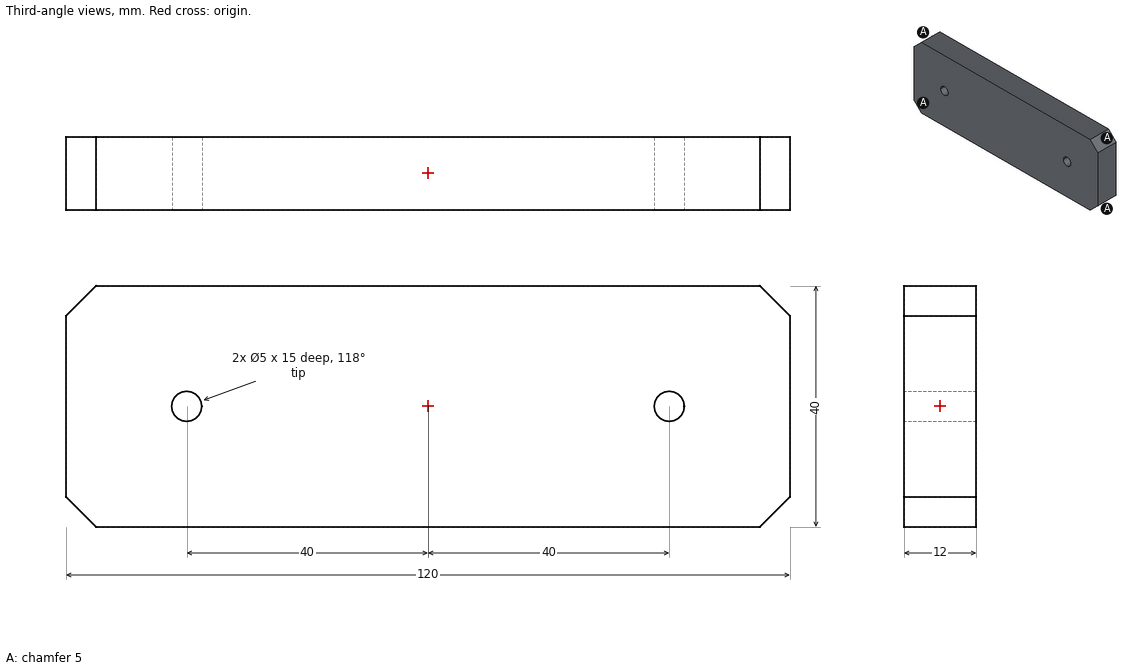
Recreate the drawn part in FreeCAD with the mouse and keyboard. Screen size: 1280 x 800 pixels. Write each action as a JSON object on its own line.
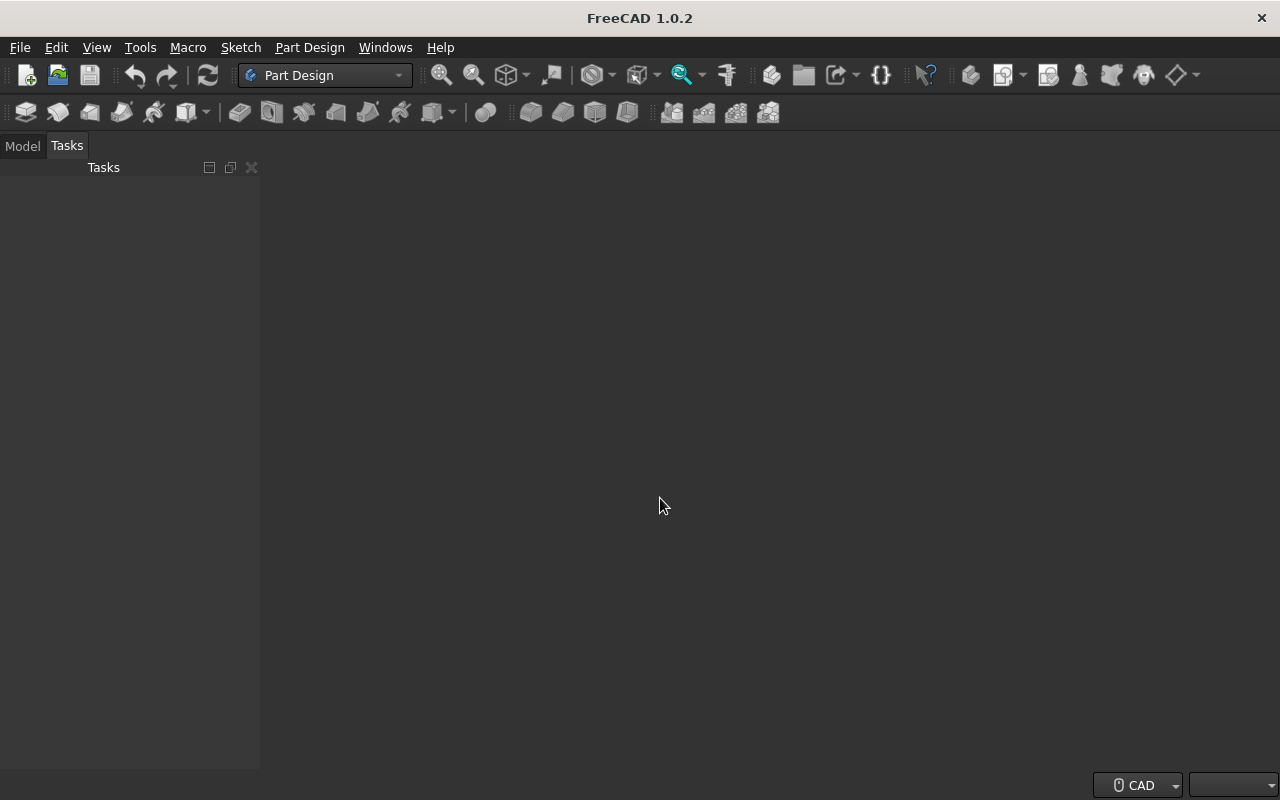
{"action": "left_click", "coordinate": [26, 76]}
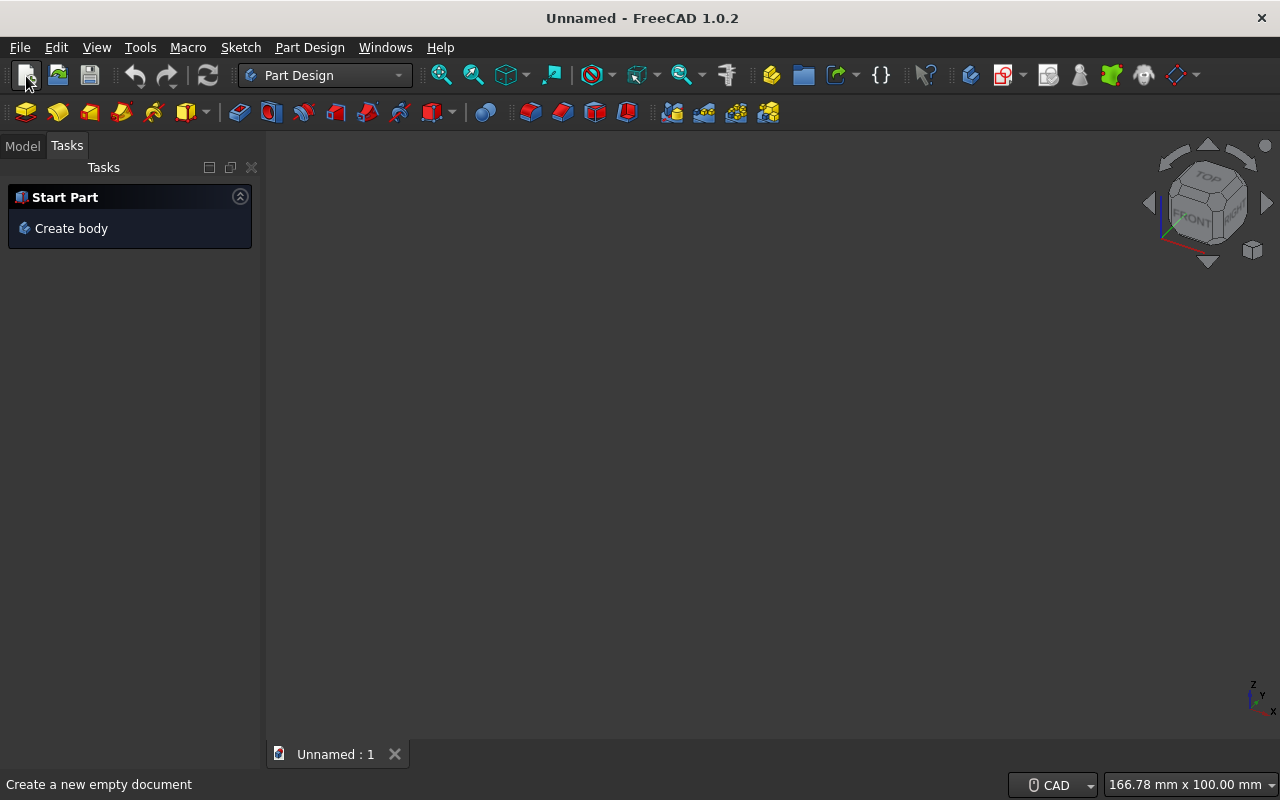
{"action": "left_click", "coordinate": [1004, 76]}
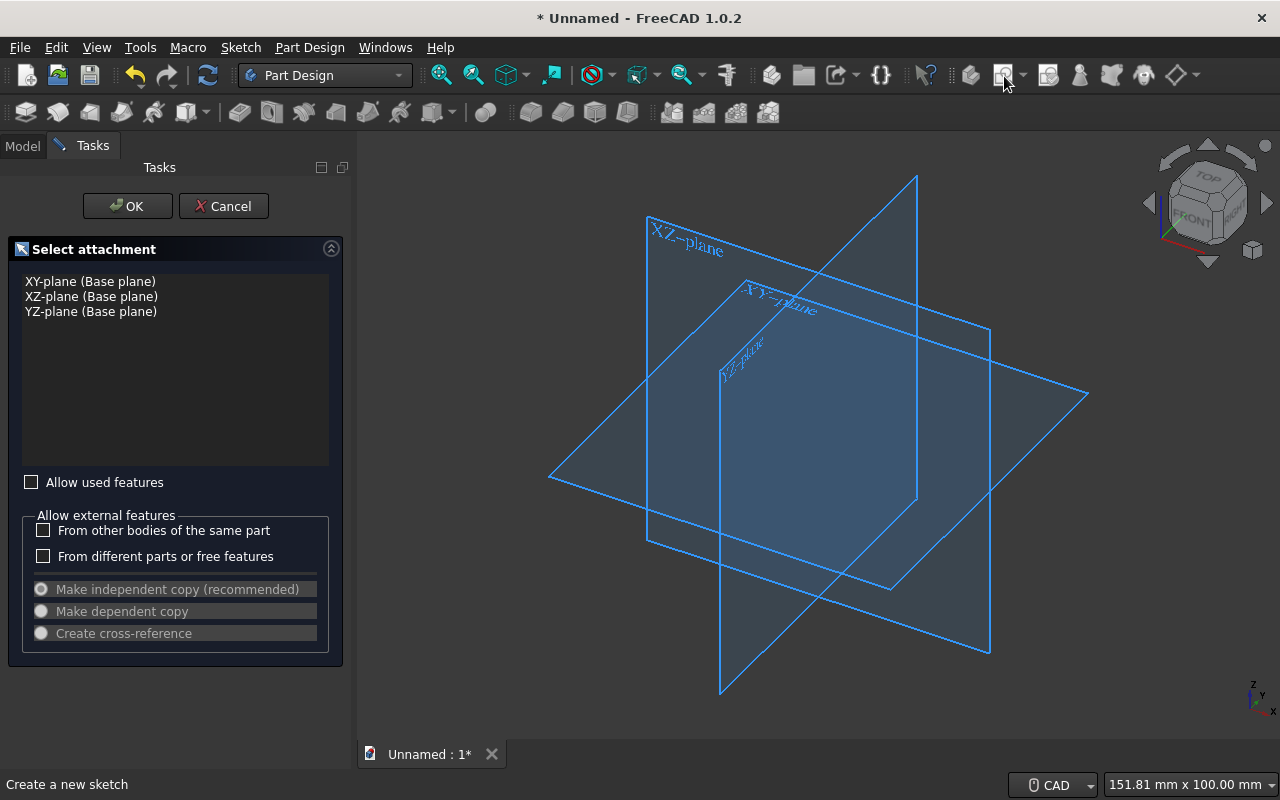
{"action": "left_click", "coordinate": [82, 296]}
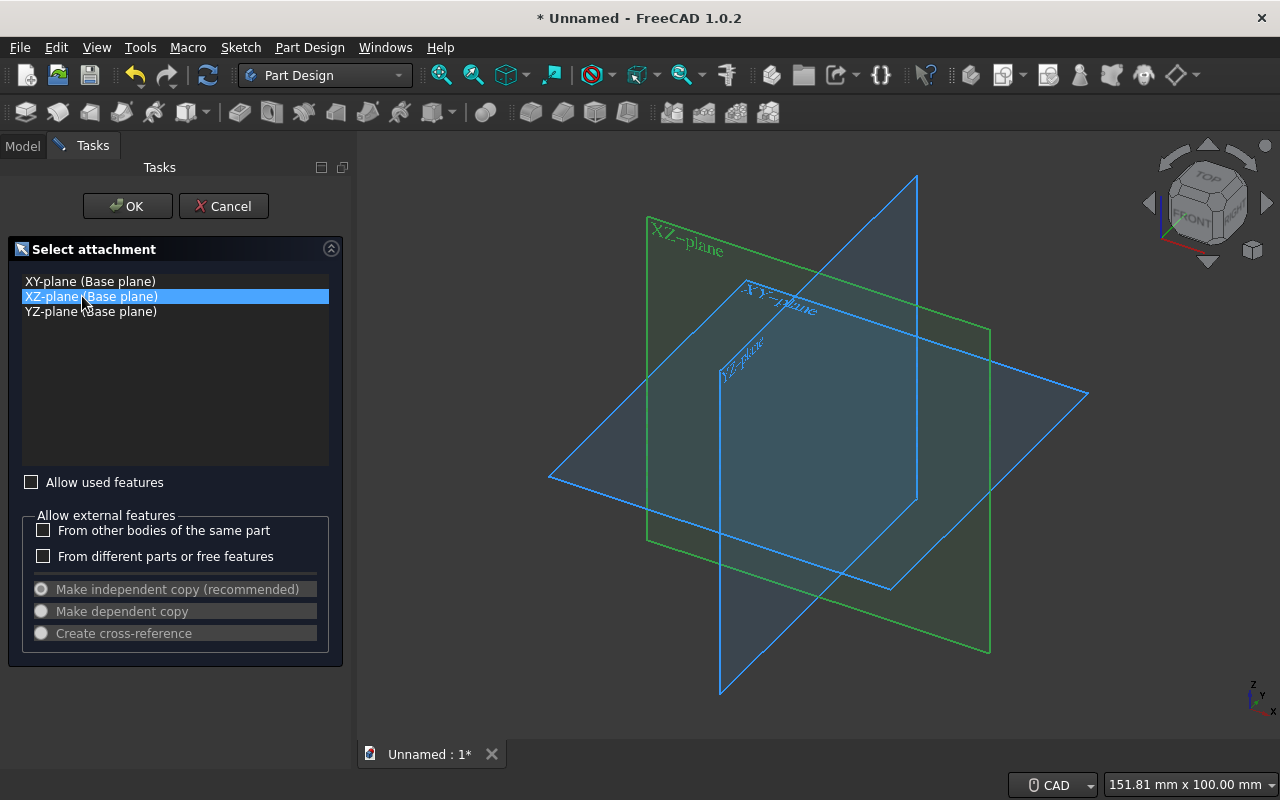
{"action": "left_click", "coordinate": [128, 206]}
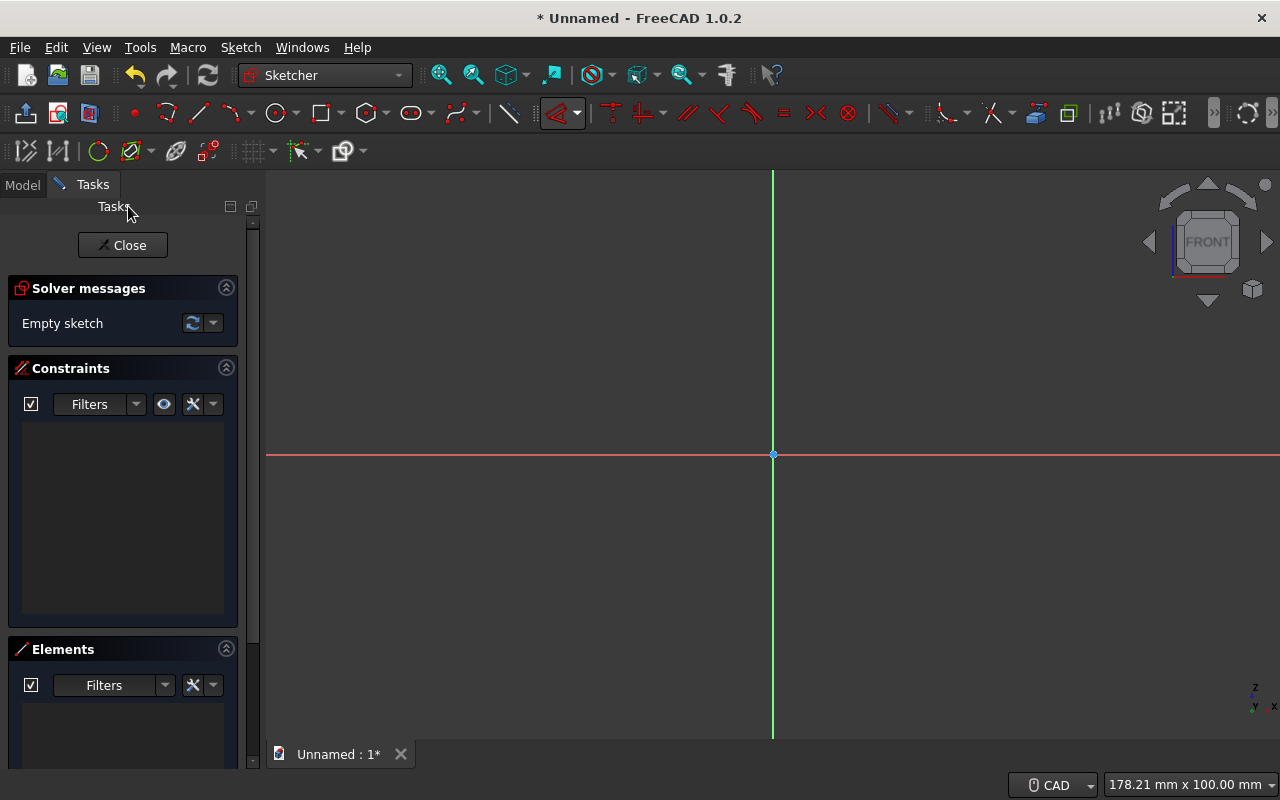
{"action": "scroll", "coordinate": [395, 455], "scroll_direction": "down", "scroll_amount": 1}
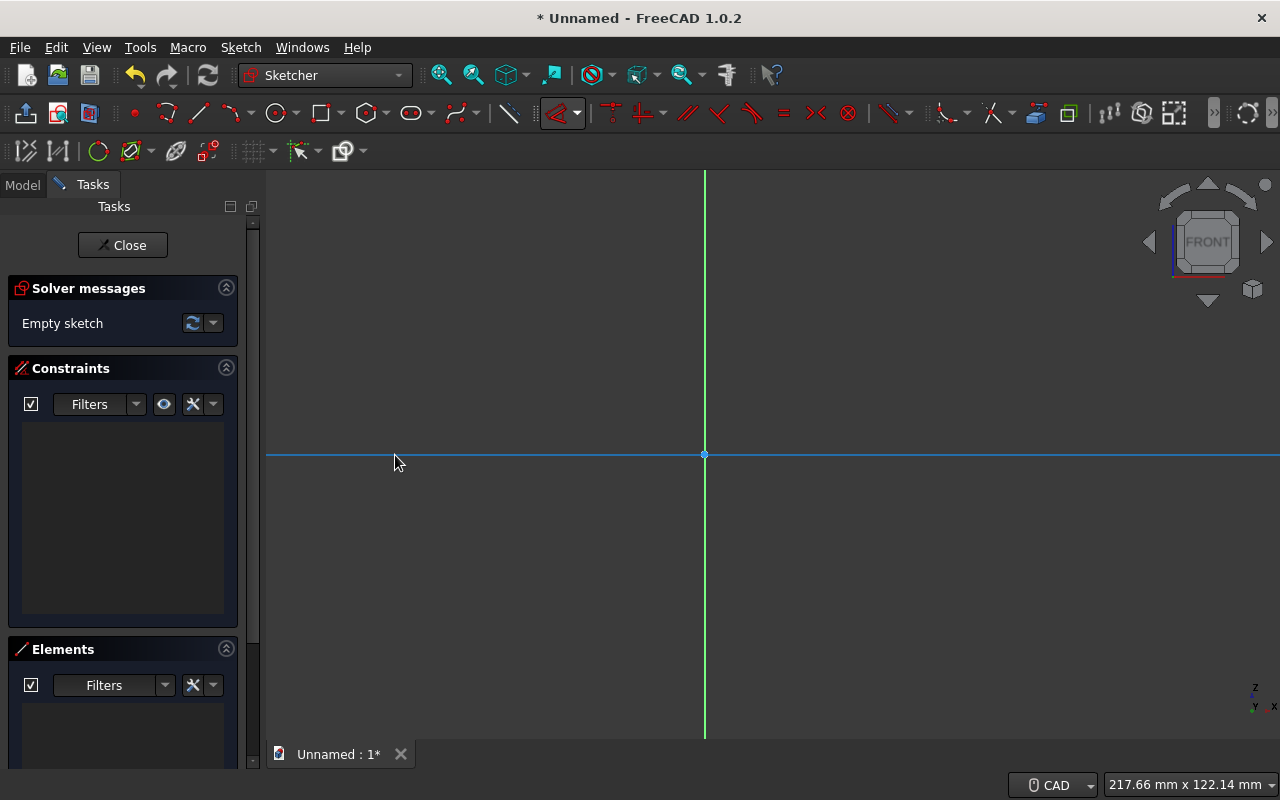
{"action": "left_click", "coordinate": [344, 114]}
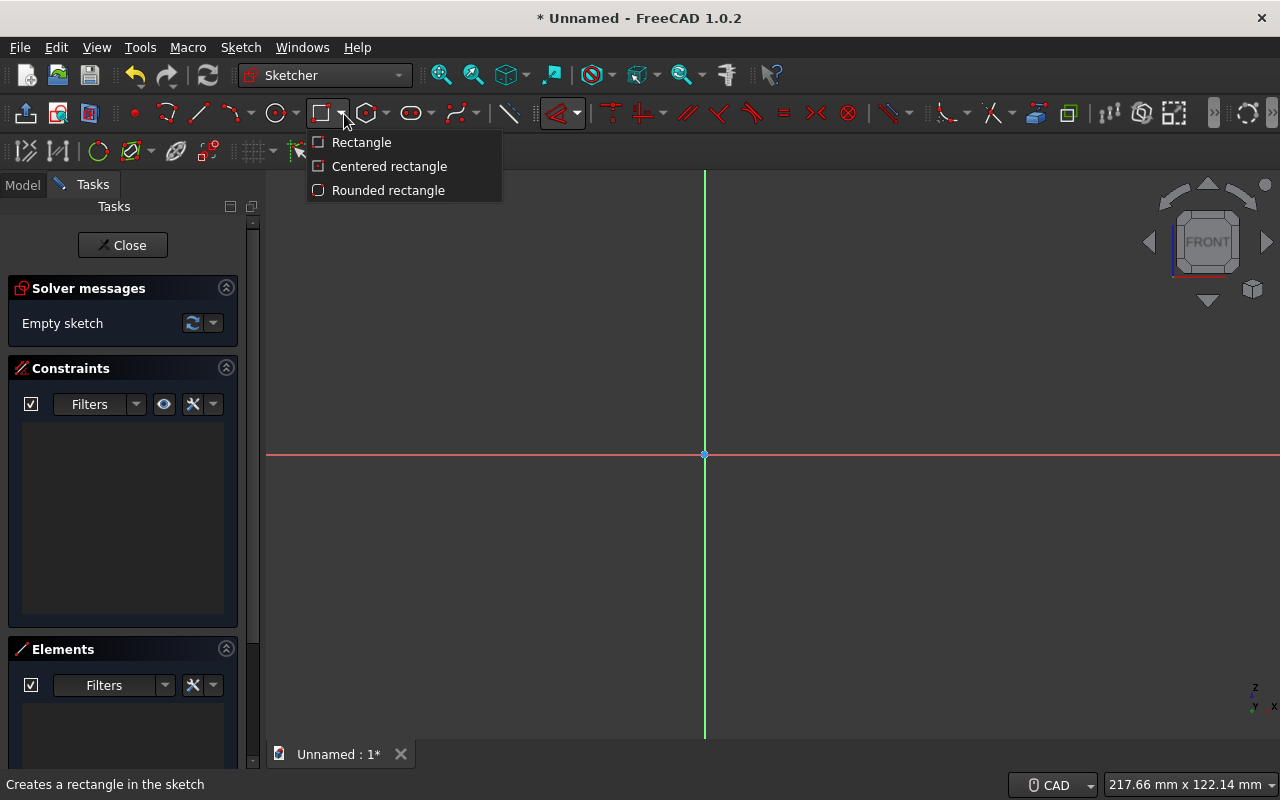
{"action": "left_click", "coordinate": [404, 166]}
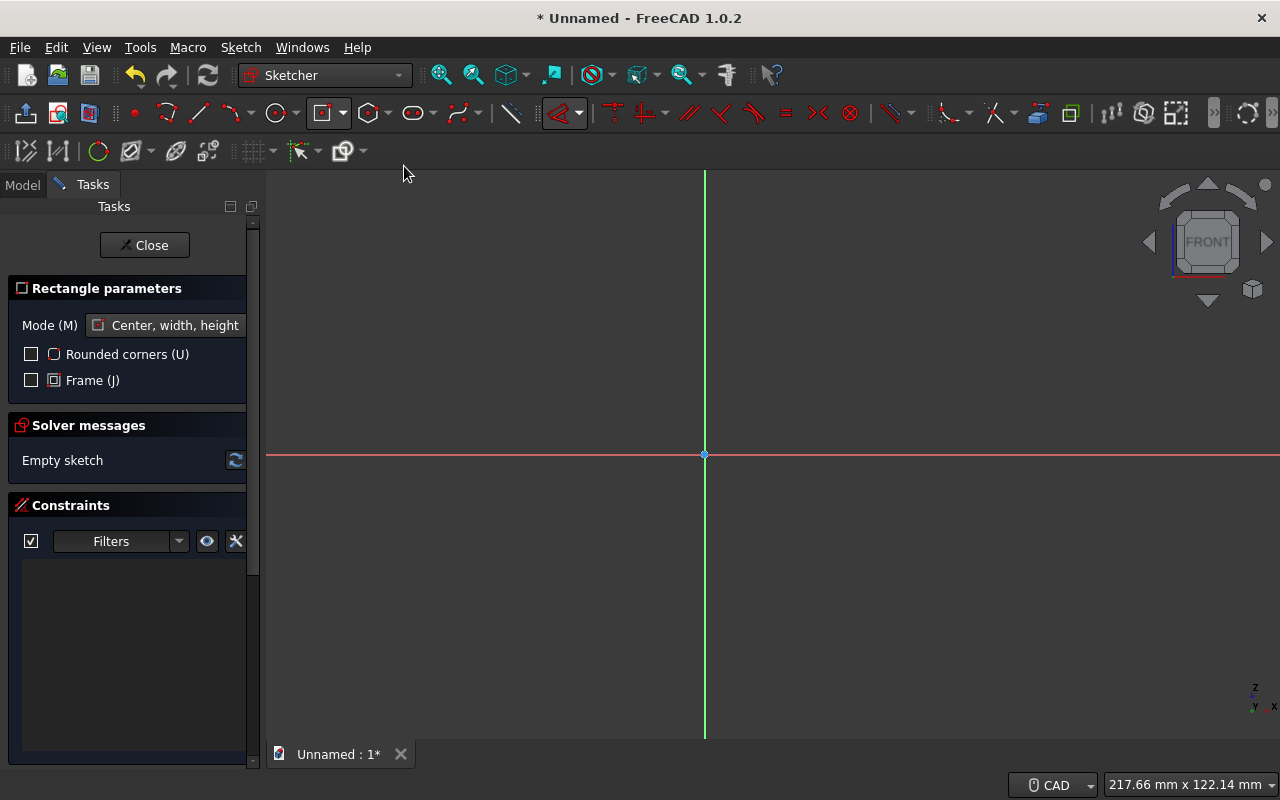
{"action": "left_click", "coordinate": [705, 455]}
{"action": "left_click", "coordinate": [984, 362]}
{"action": "key", "text": "Escape"}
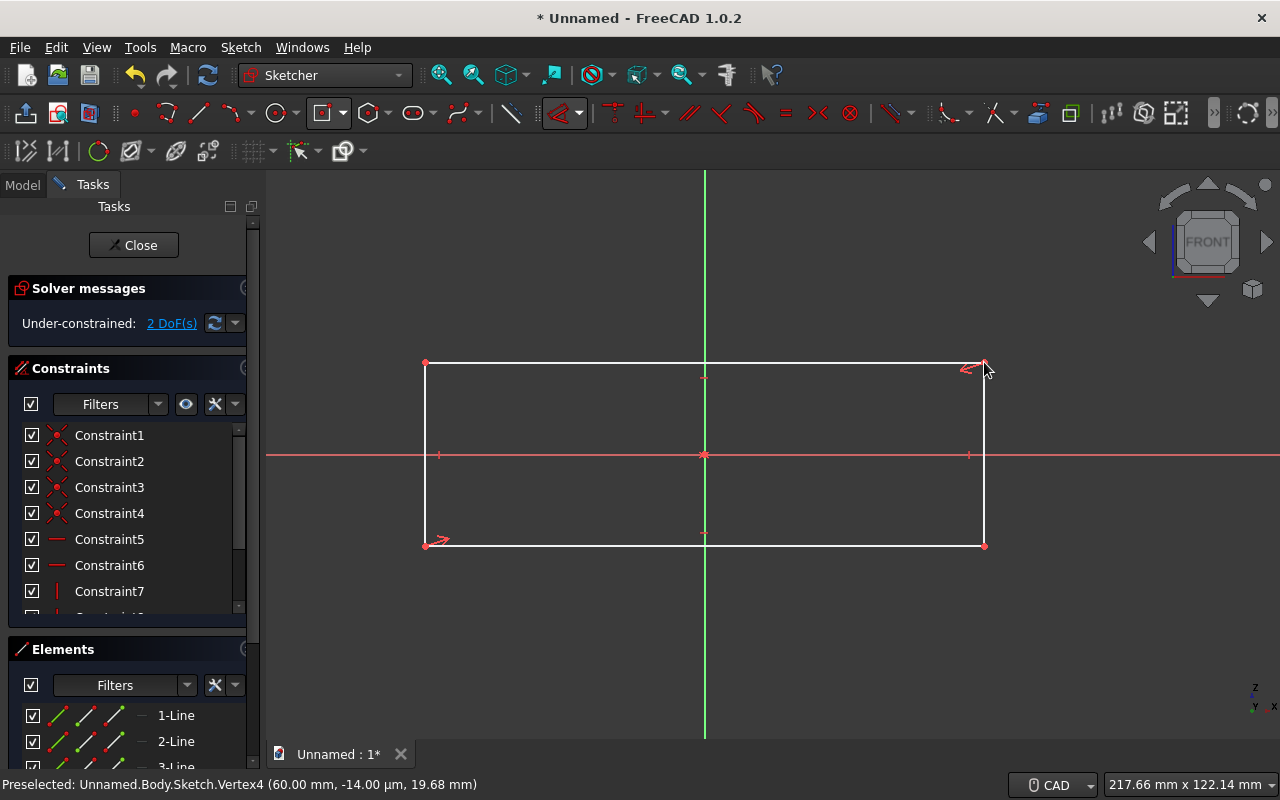
{"action": "left_click", "coordinate": [558, 114]}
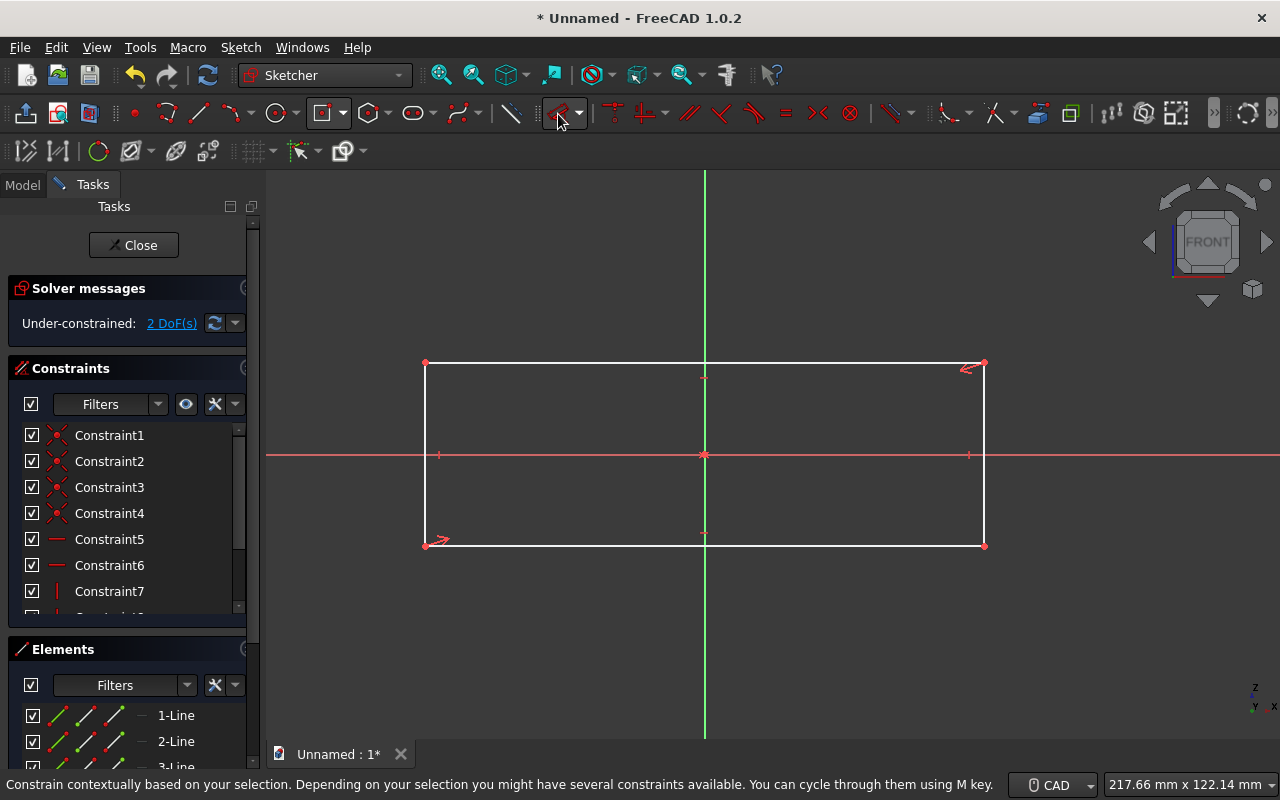
{"action": "left_click", "coordinate": [984, 491]}
{"action": "left_click", "coordinate": [1018, 413]}